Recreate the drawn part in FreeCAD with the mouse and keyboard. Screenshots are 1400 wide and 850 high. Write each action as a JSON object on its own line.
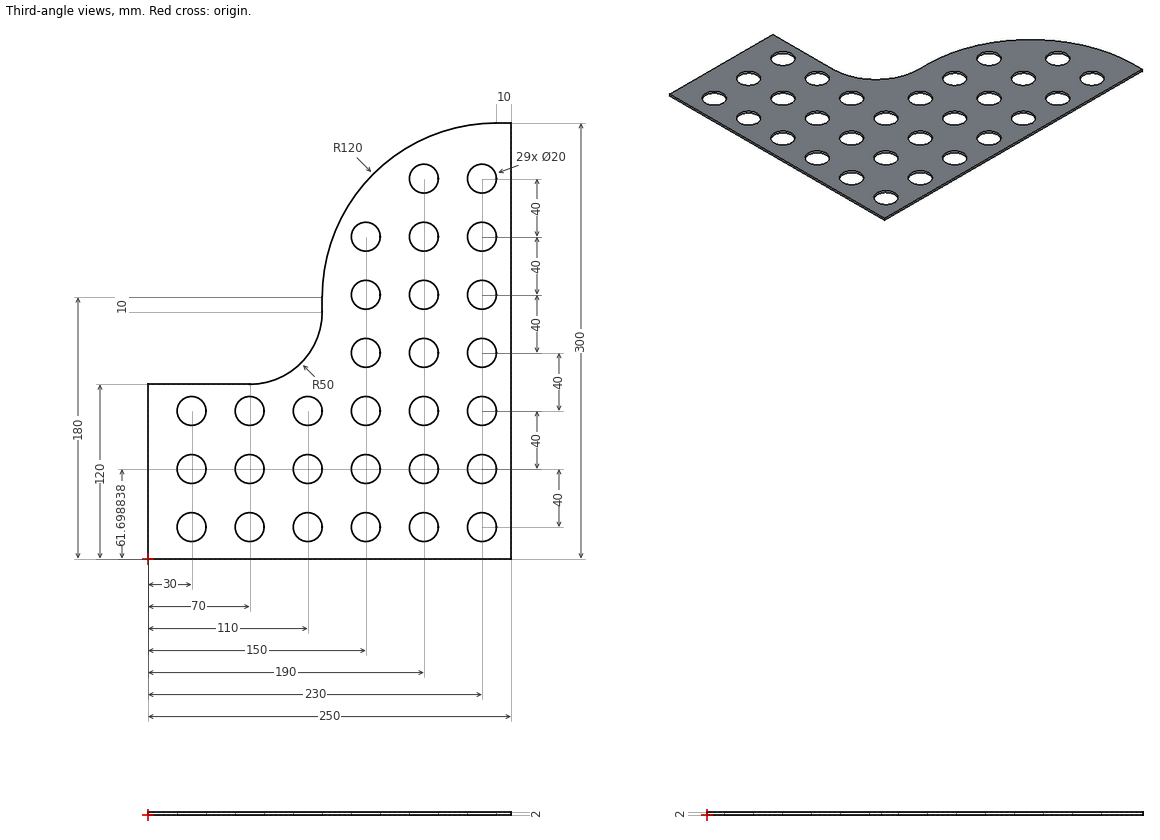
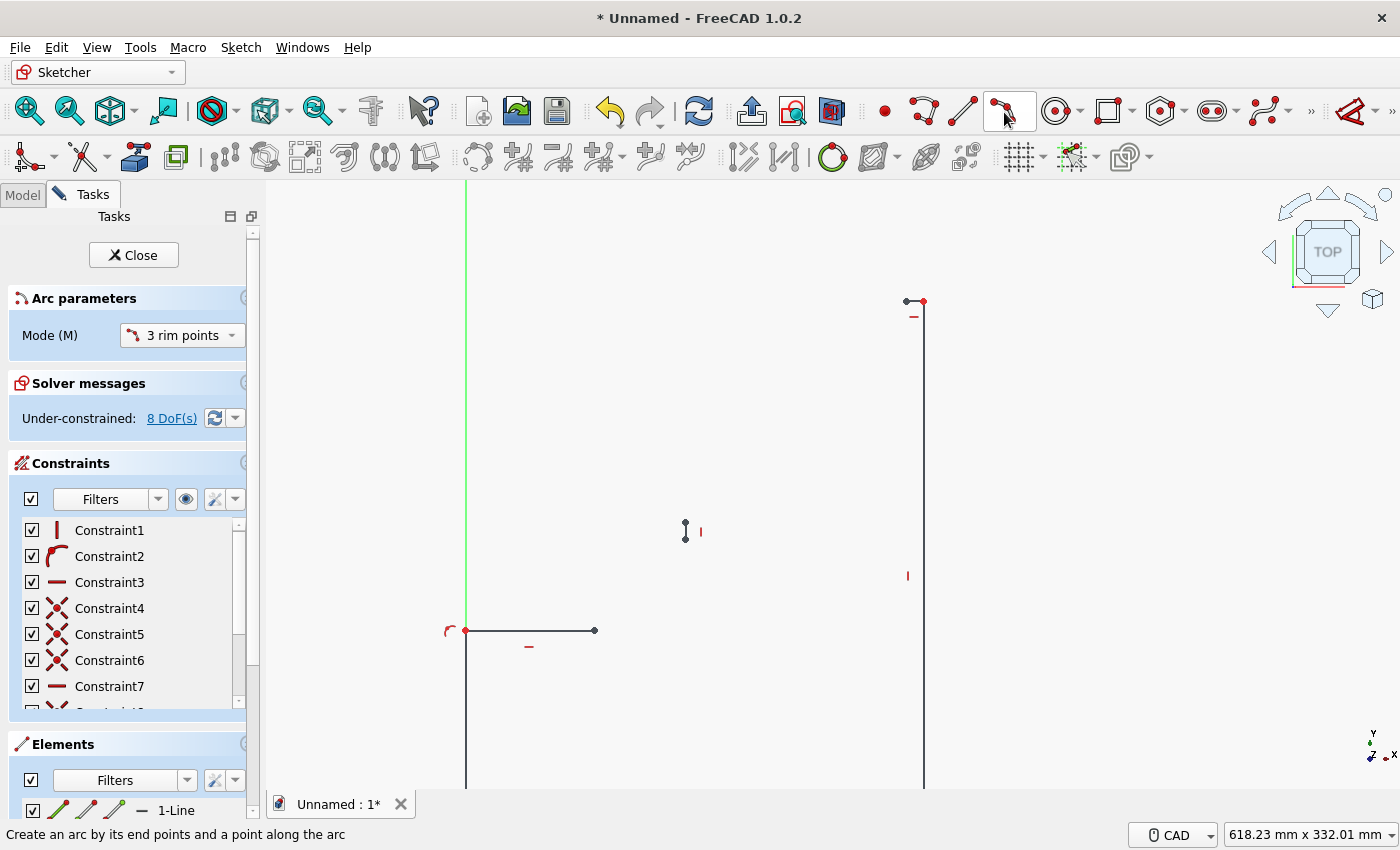
{"action": "scroll", "coordinate": [686, 539], "scroll_direction": "up", "scroll_amount": 3}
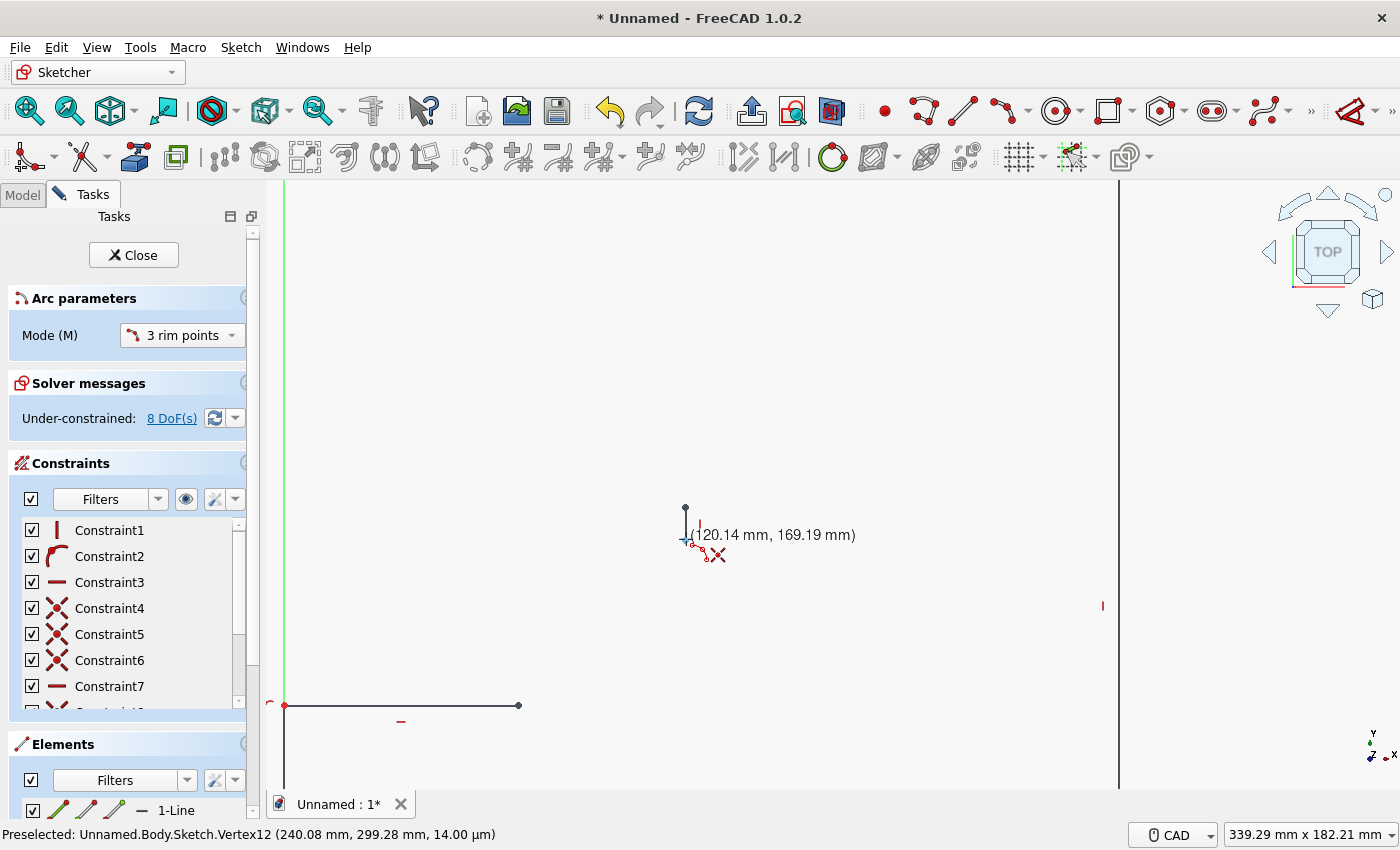
{"action": "left_click", "coordinate": [686, 540]}
{"action": "left_click", "coordinate": [518, 706]}
{"action": "left_click", "coordinate": [636, 656]}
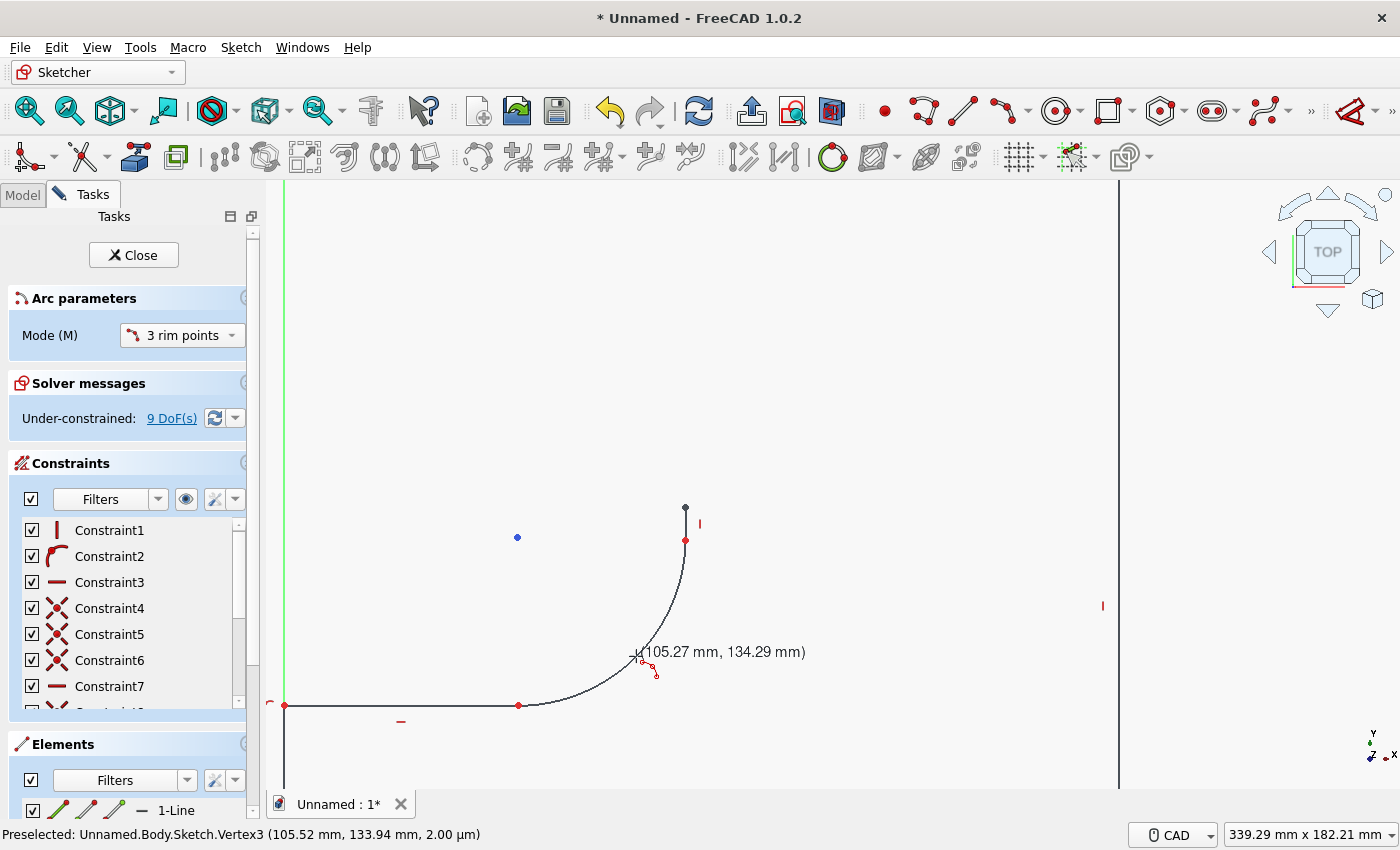
{"action": "scroll", "coordinate": [801, 415], "scroll_direction": "down", "scroll_amount": 5}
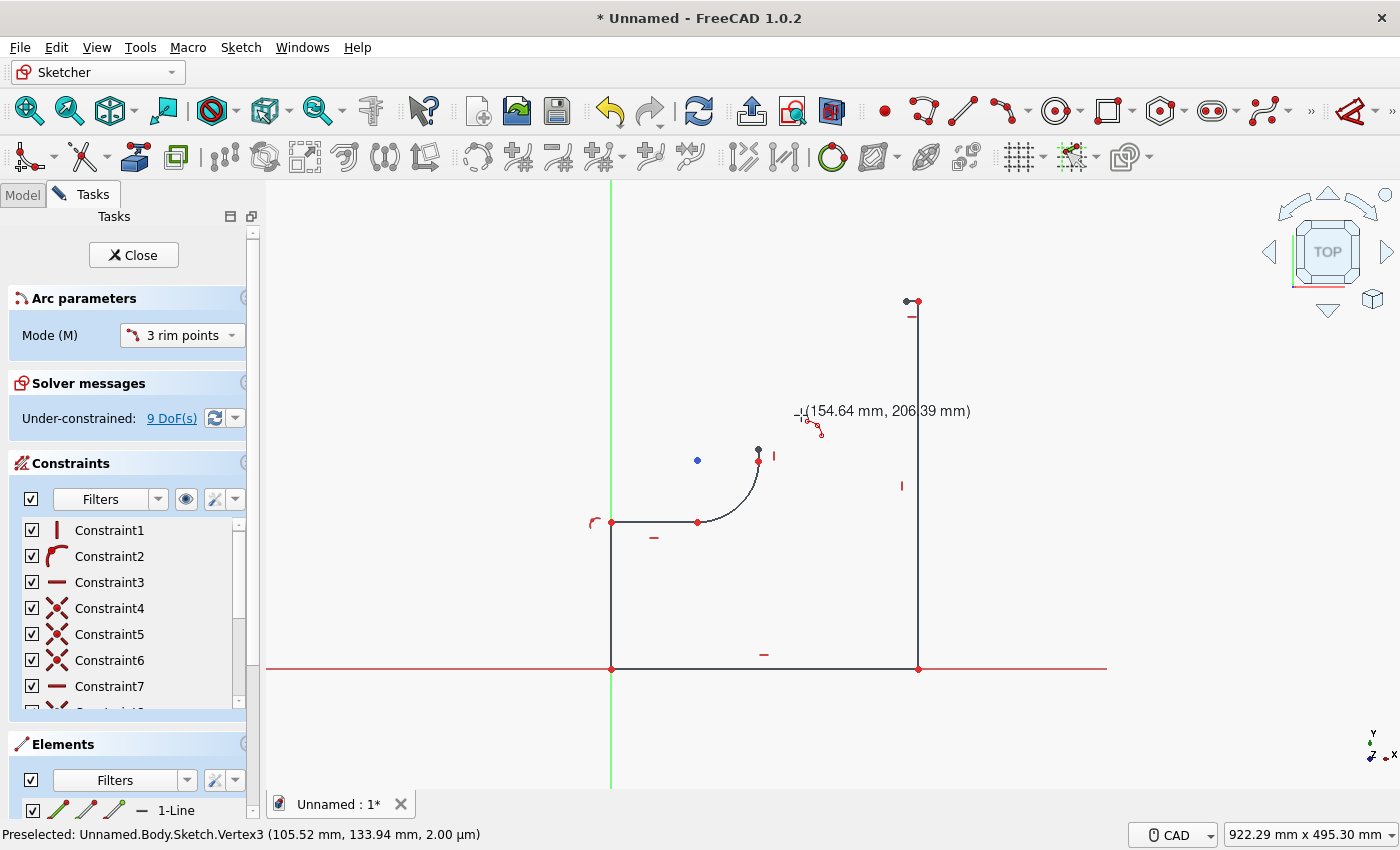
{"action": "scroll", "coordinate": [906, 301], "scroll_direction": "up", "scroll_amount": 5}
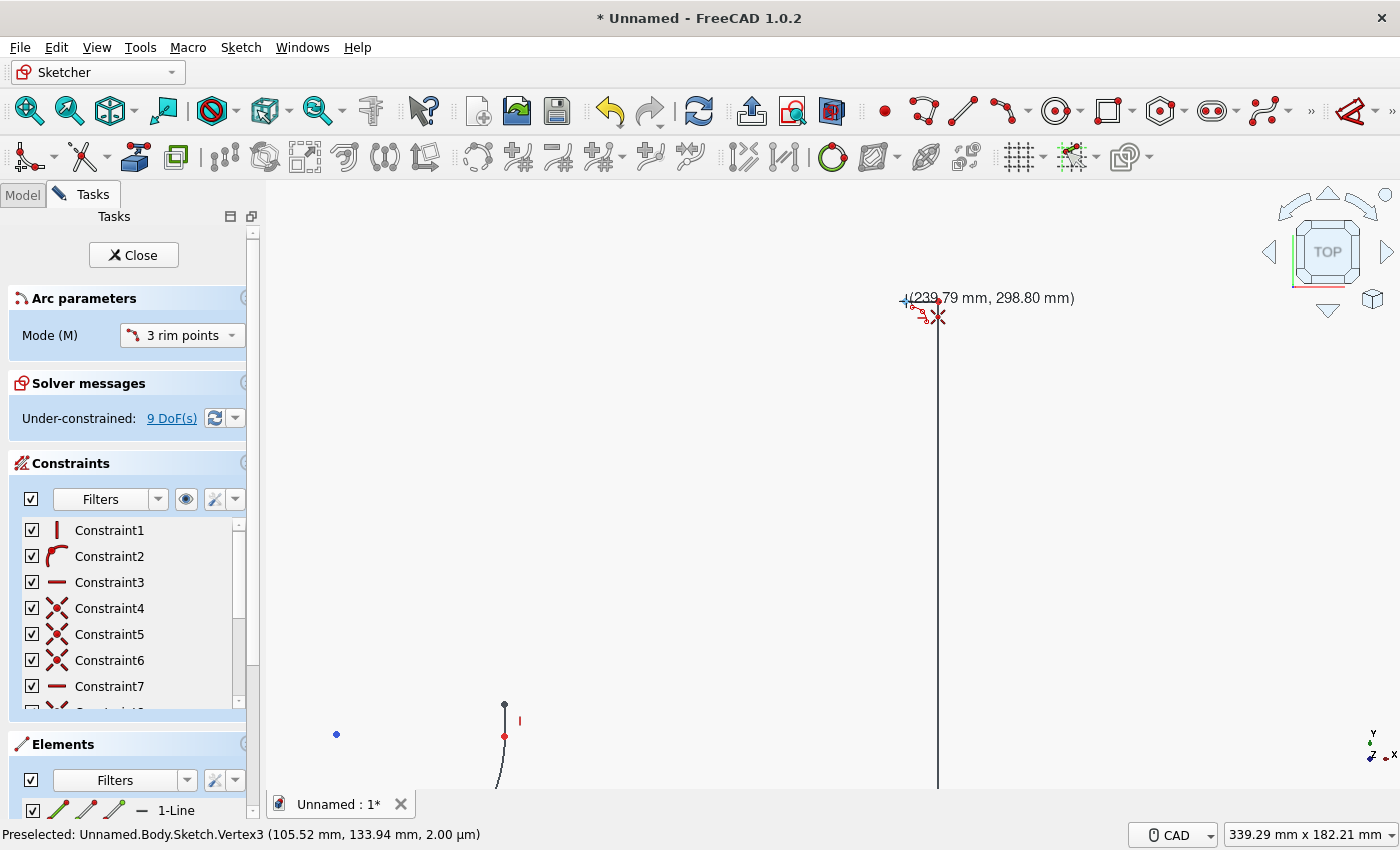
{"action": "left_click", "coordinate": [906, 302]}
{"action": "left_click", "coordinate": [505, 704]}
{"action": "left_click", "coordinate": [622, 417]}
{"action": "key", "text": "Escape"}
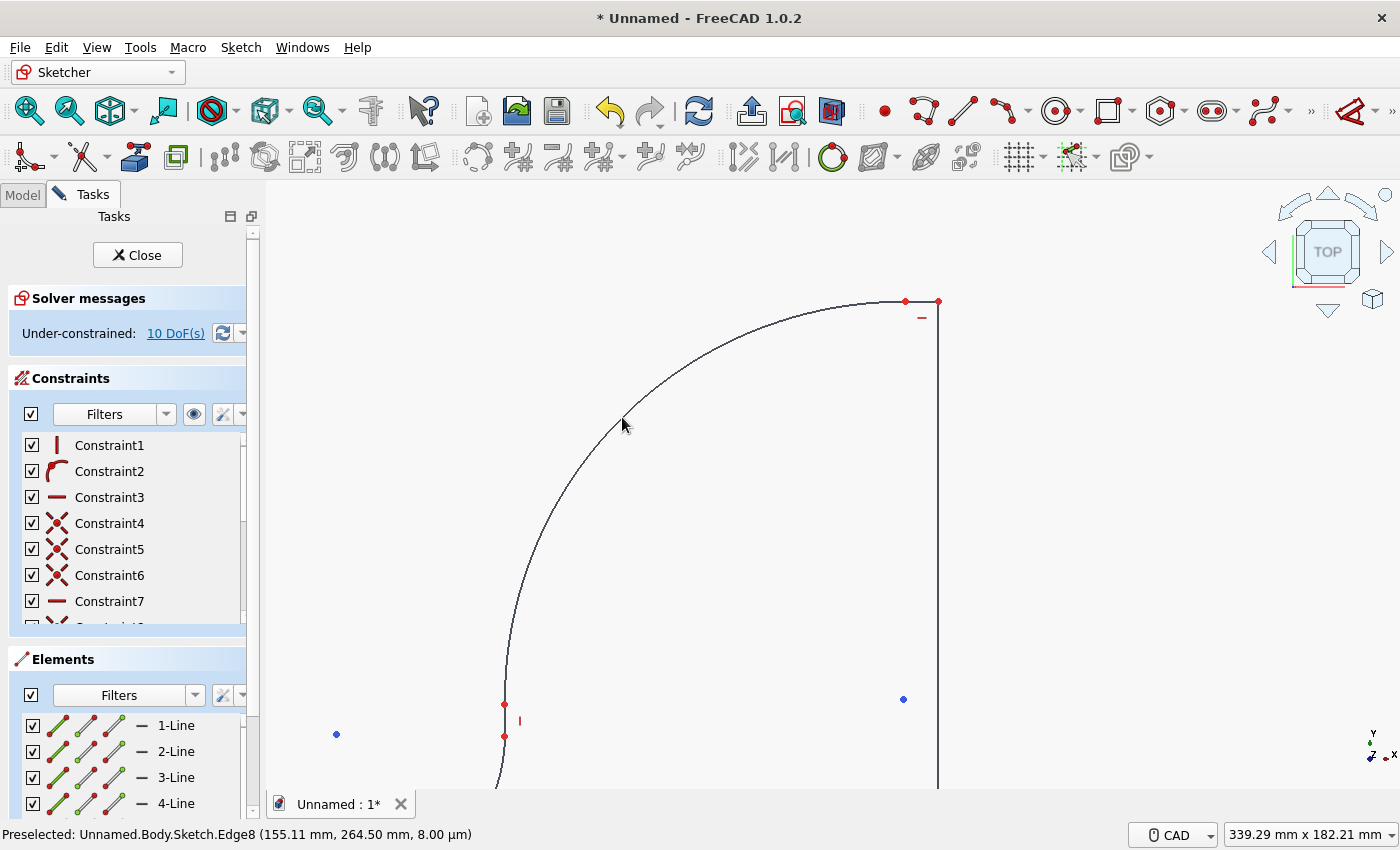
{"action": "left_click", "coordinate": [1350, 112]}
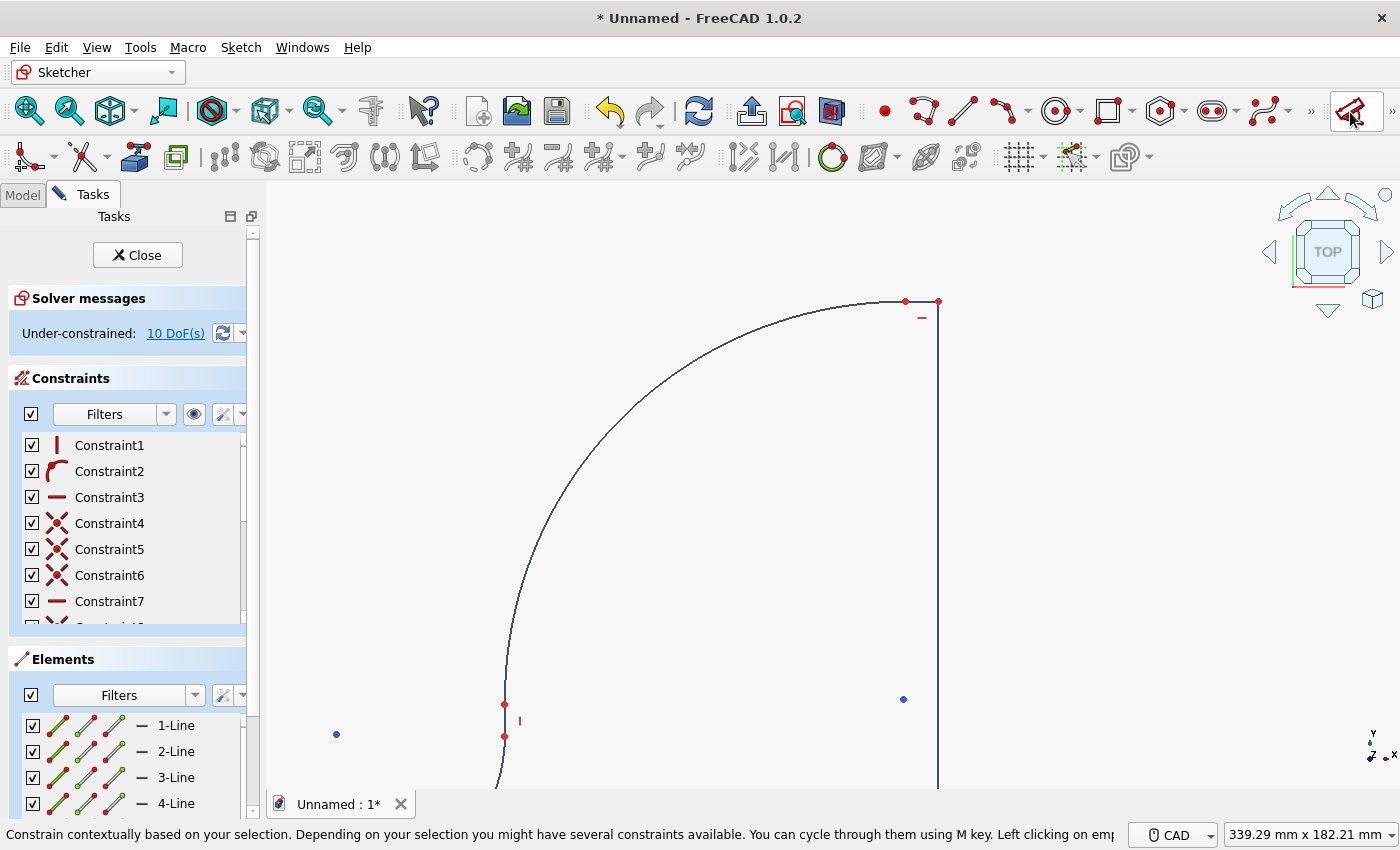
{"action": "scroll", "coordinate": [906, 300], "scroll_direction": "down", "scroll_amount": 5}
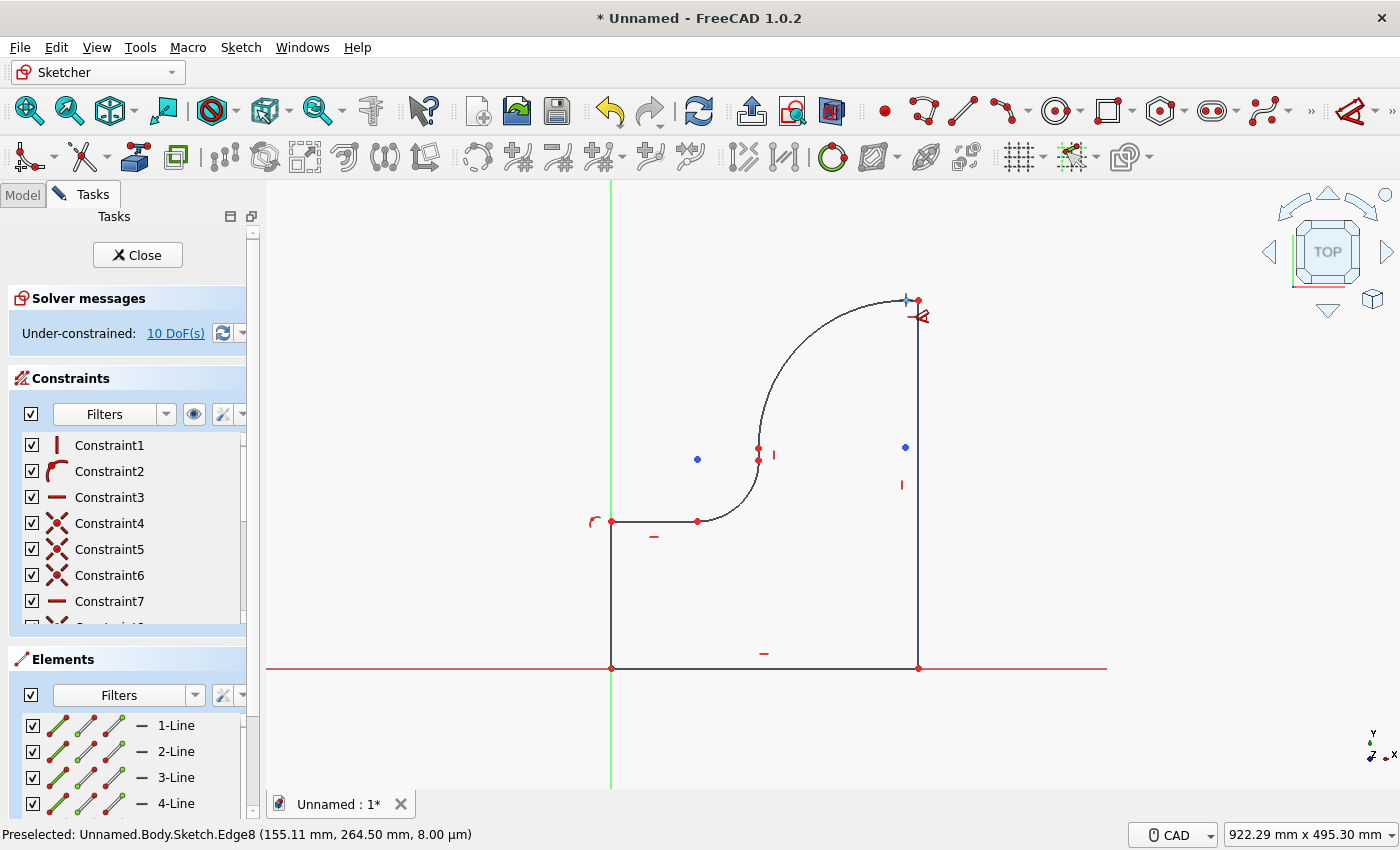
{"action": "left_click", "coordinate": [725, 515]}
{"action": "left_click", "coordinate": [739, 544]}